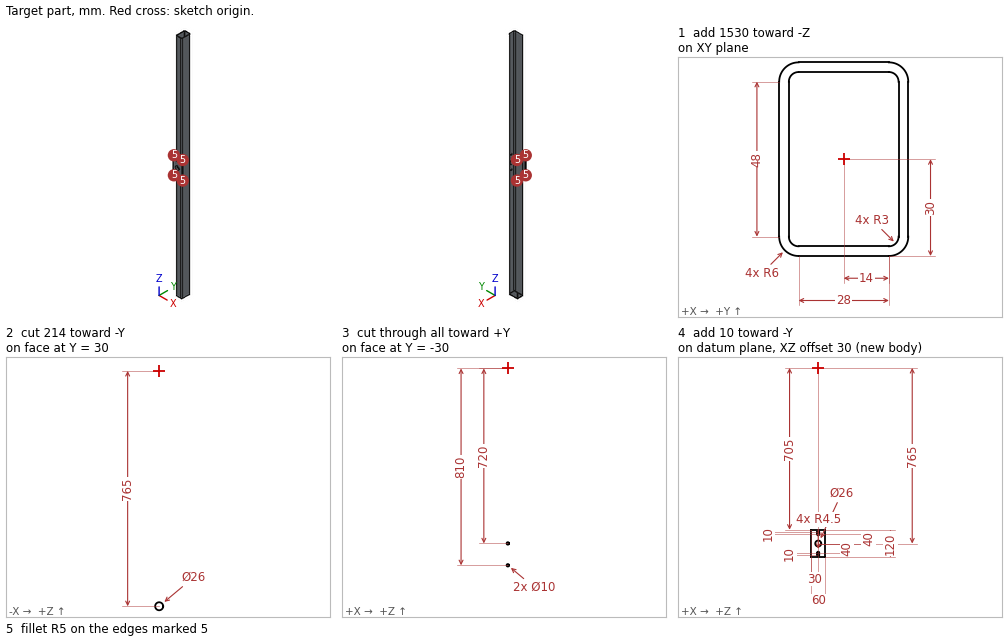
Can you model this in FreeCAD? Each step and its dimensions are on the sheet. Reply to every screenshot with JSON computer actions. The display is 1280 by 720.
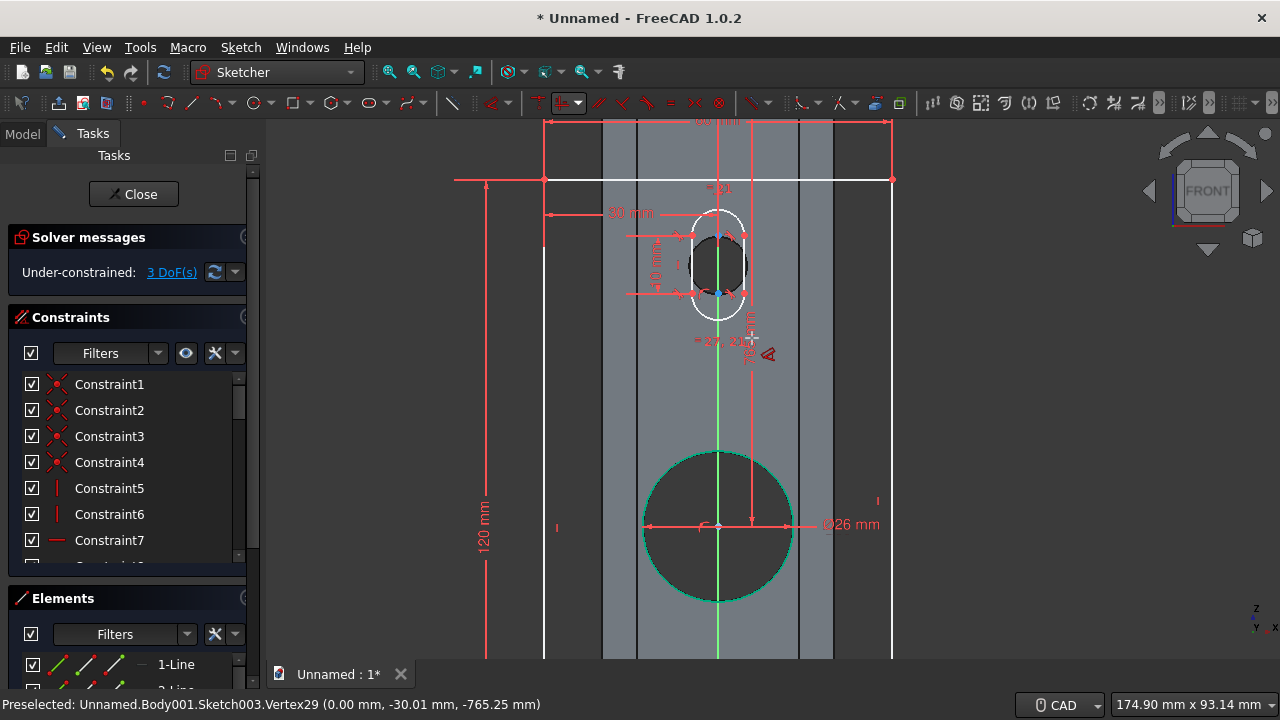
{"action": "scroll", "coordinate": [693, 277], "scroll_direction": "down", "scroll_amount": 4}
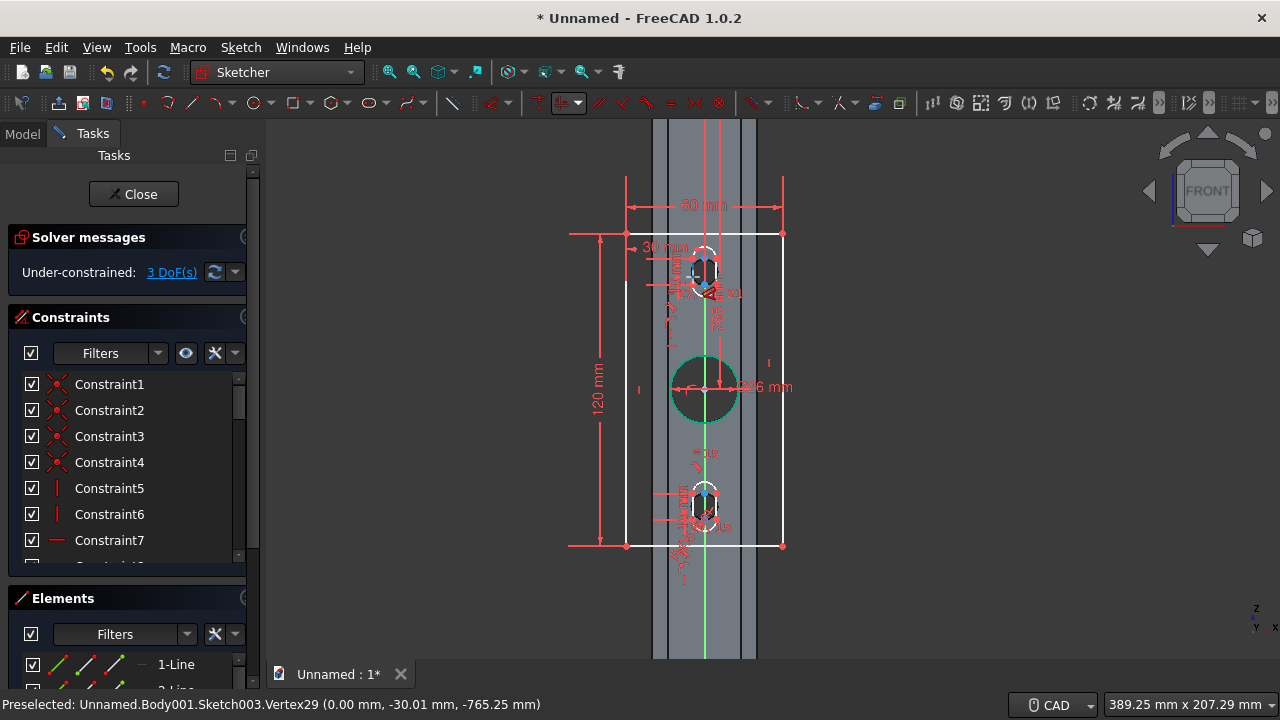
{"action": "left_click", "coordinate": [716, 494]}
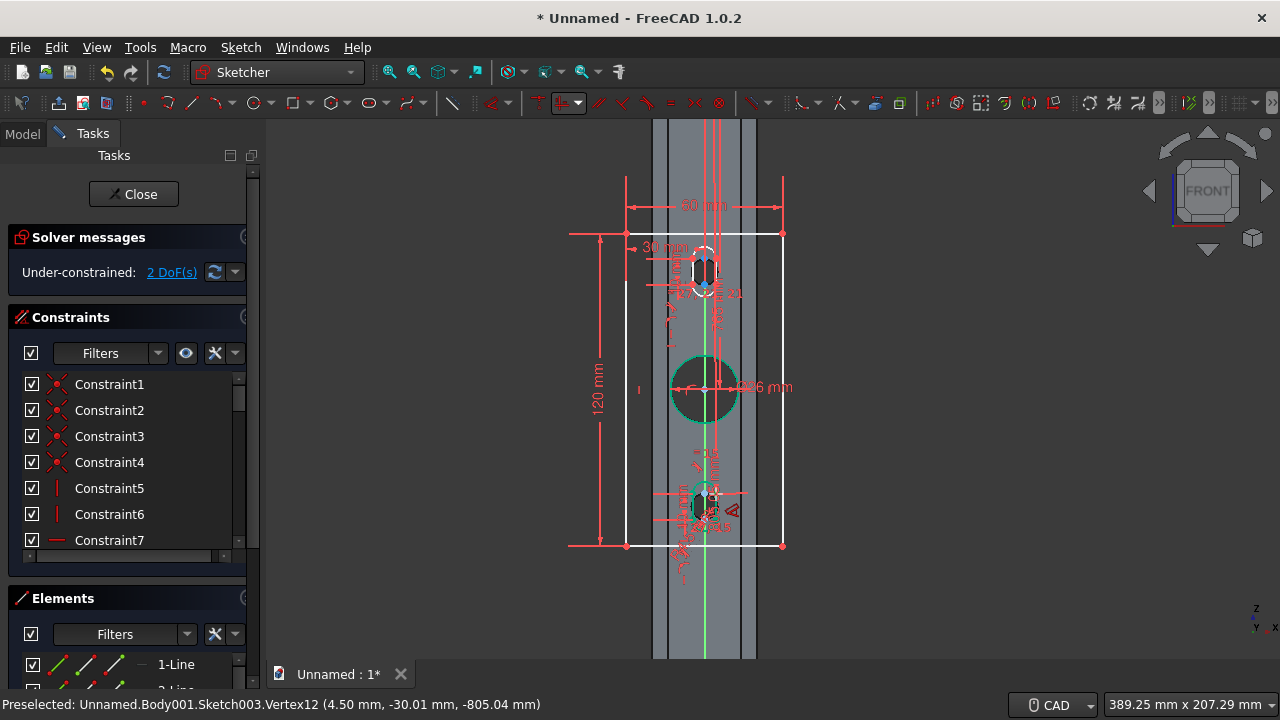
{"action": "left_click", "coordinate": [705, 389]}
{"action": "left_click", "coordinate": [750, 441]}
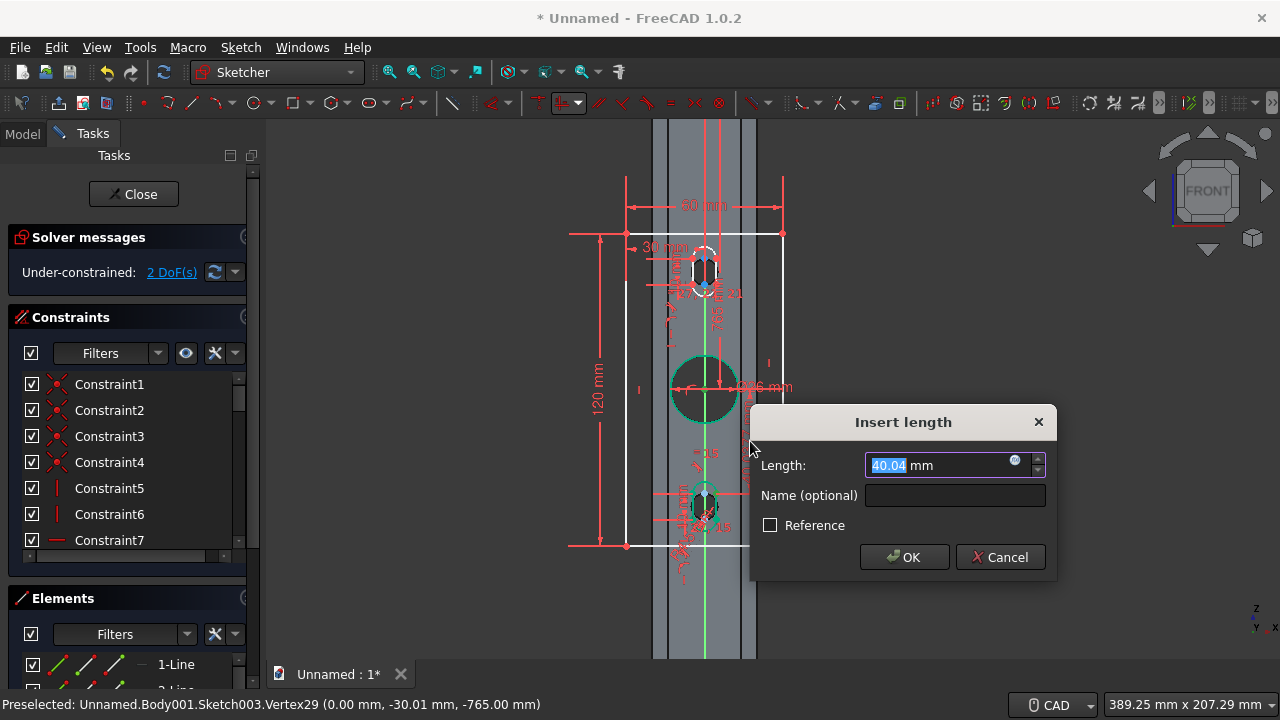
{"action": "type", "text": "40"}
{"action": "key", "text": "Return"}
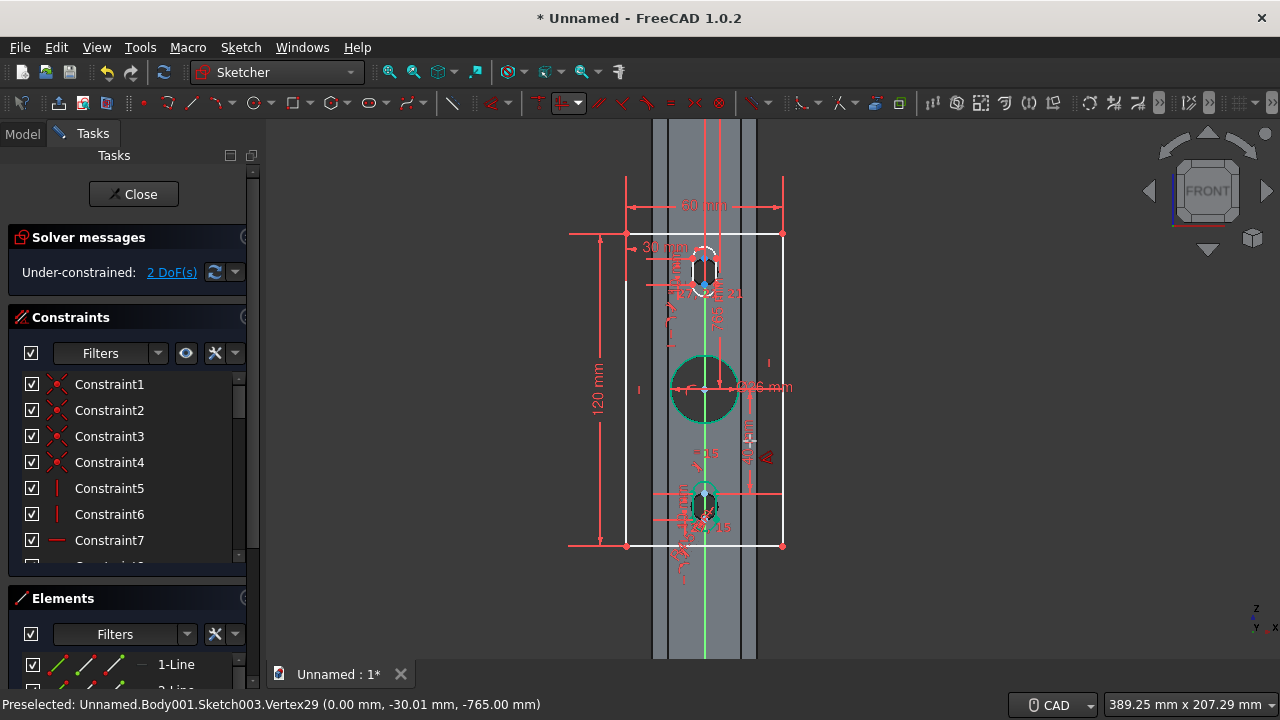
{"action": "left_click", "coordinate": [693, 285]}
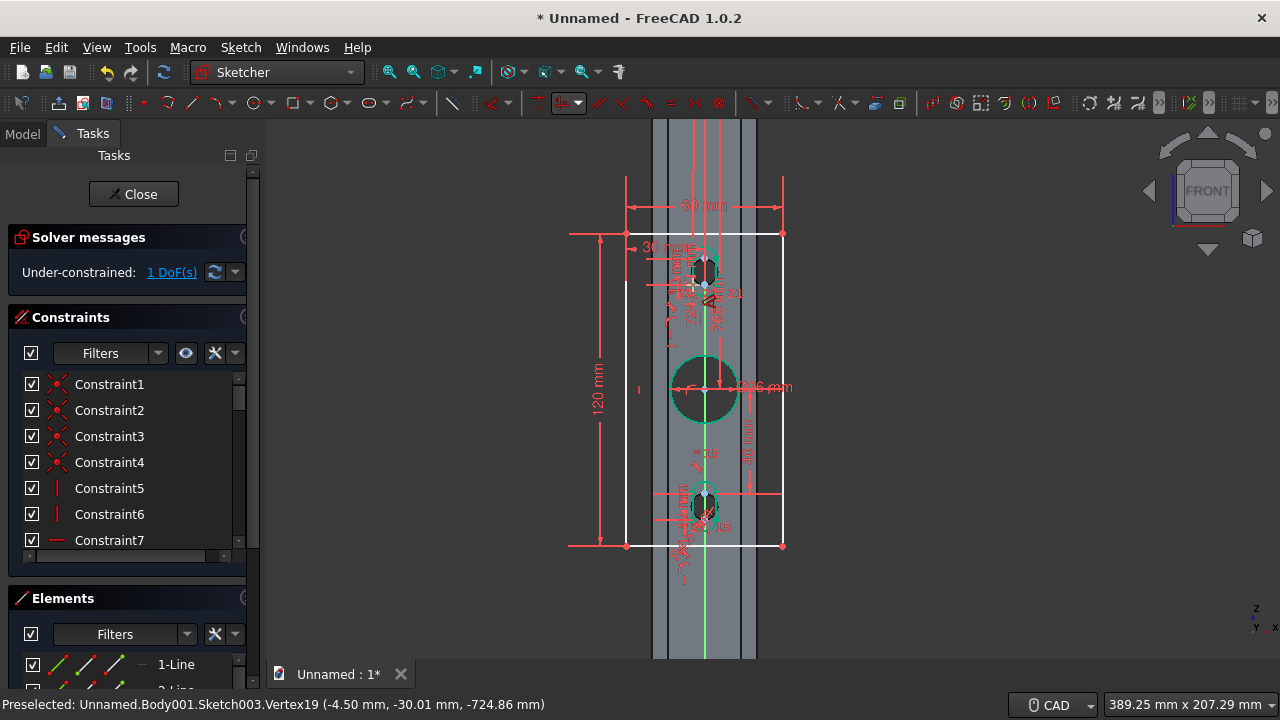
{"action": "left_click", "coordinate": [705, 389]}
{"action": "left_click", "coordinate": [659, 337]}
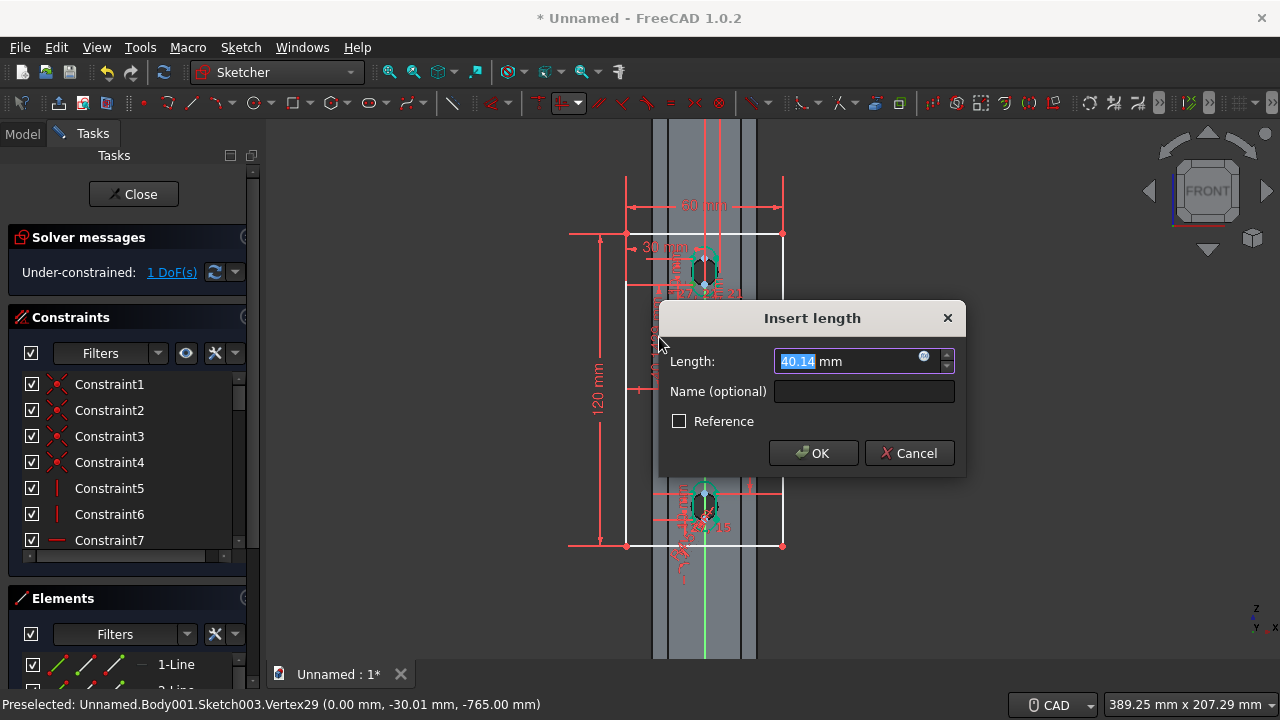
{"action": "type", "text": "40"}
{"action": "key", "text": "Return"}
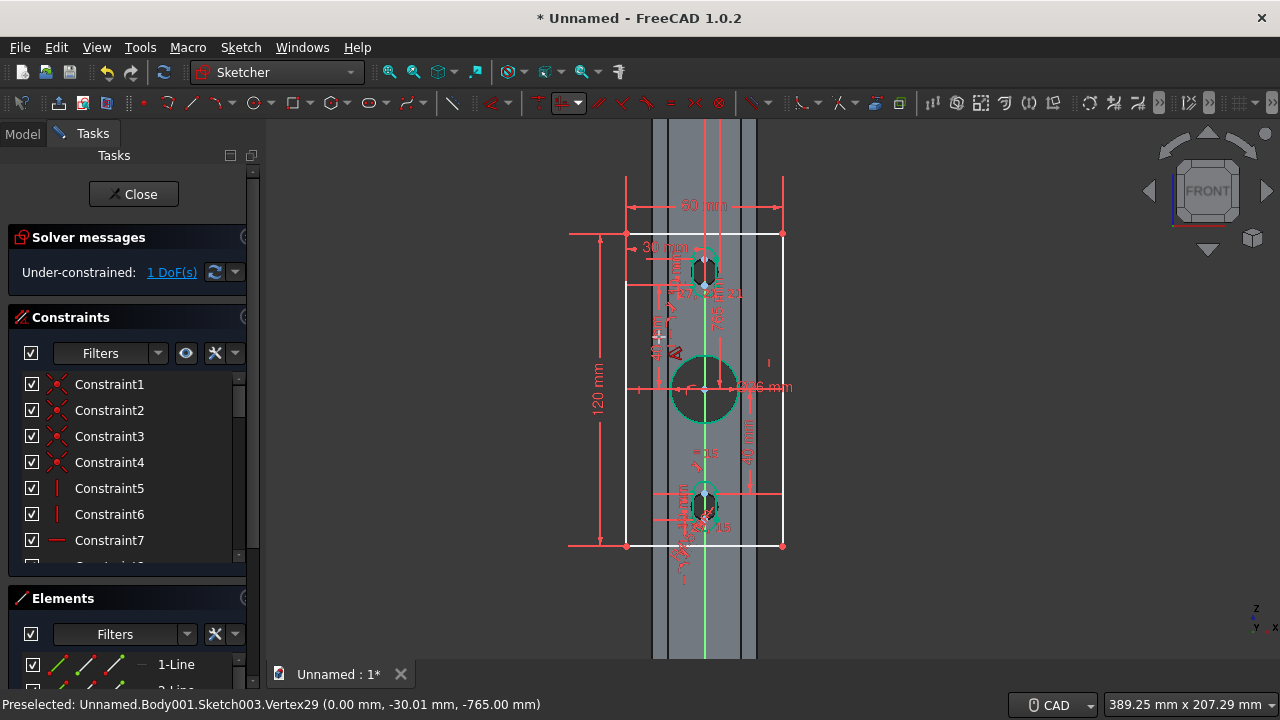
{"action": "left_click", "coordinate": [626, 234]}
{"action": "left_click", "coordinate": [592, 190]}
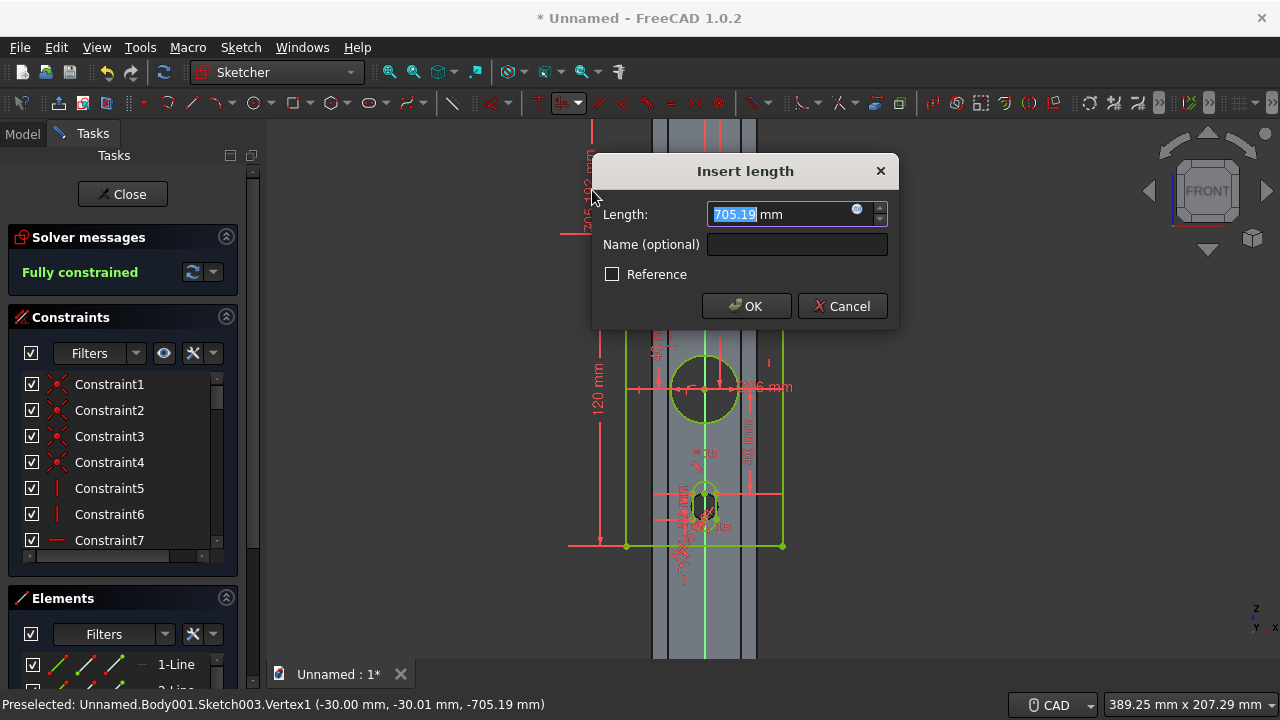
{"action": "type", "text": "705"}
{"action": "key", "text": "Return"}
{"action": "key", "text": "Escape"}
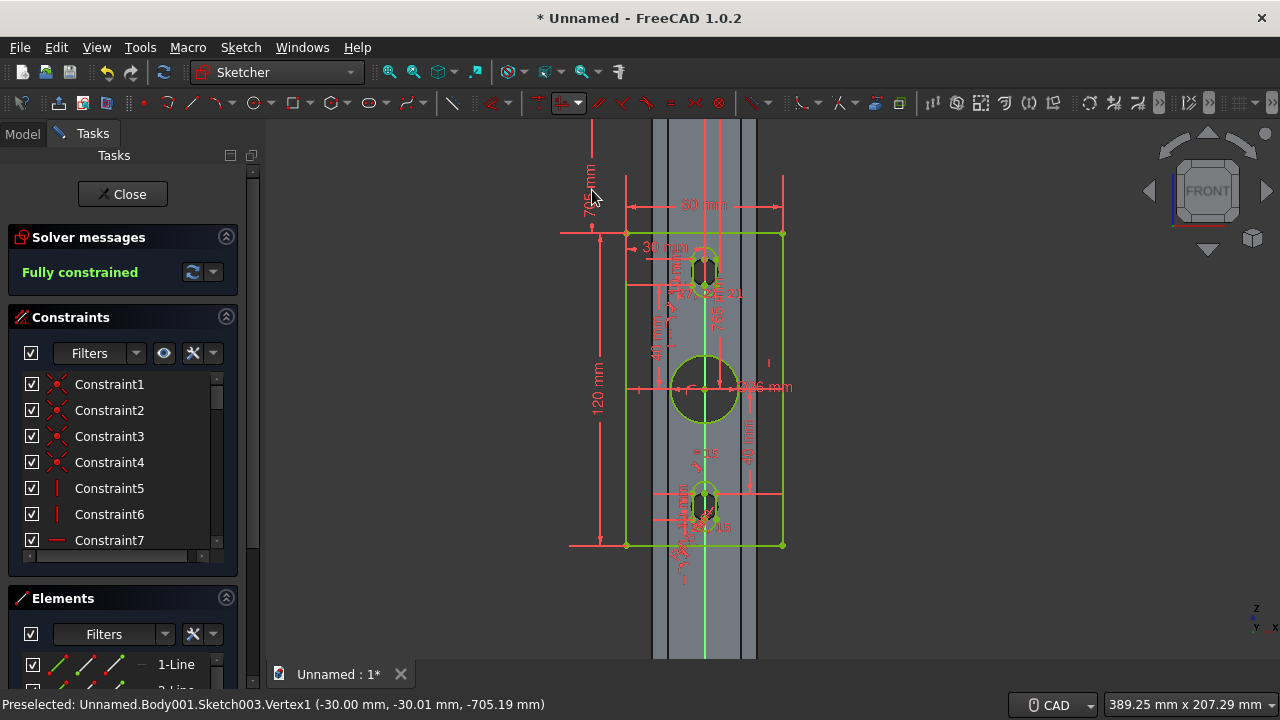
{"action": "left_click", "coordinate": [123, 194]}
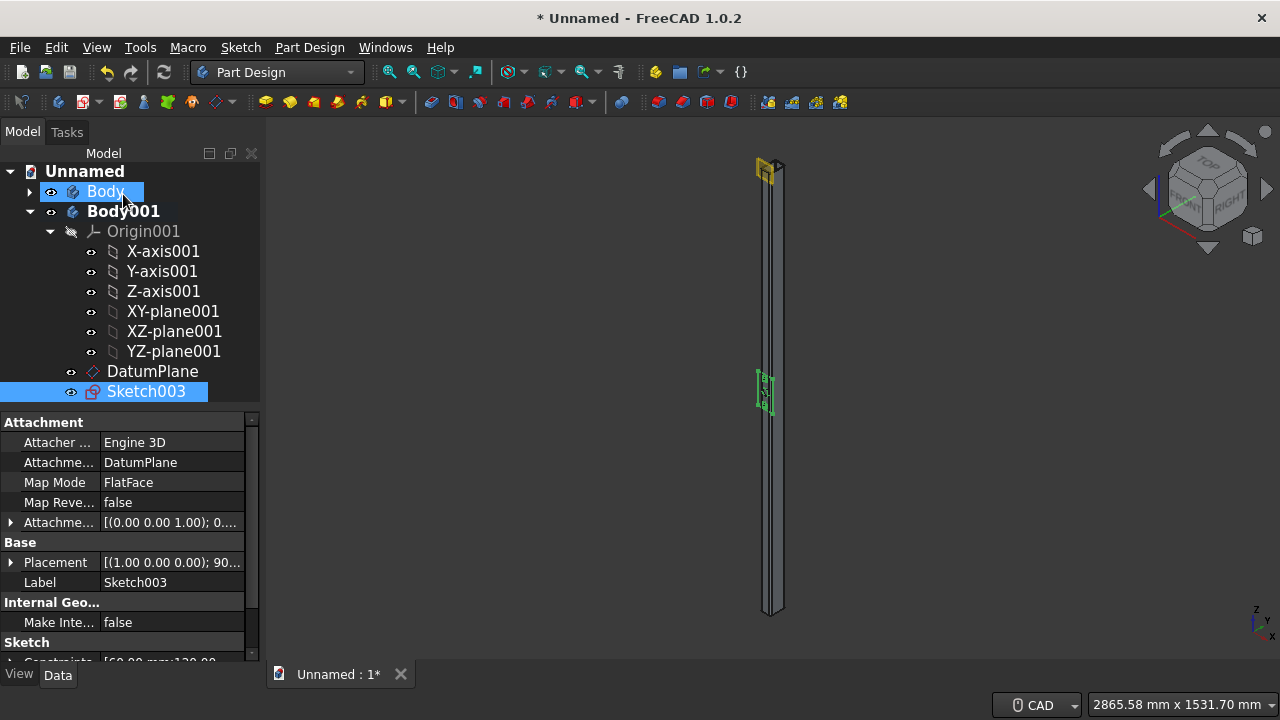
{"action": "left_click", "coordinate": [266, 102]}